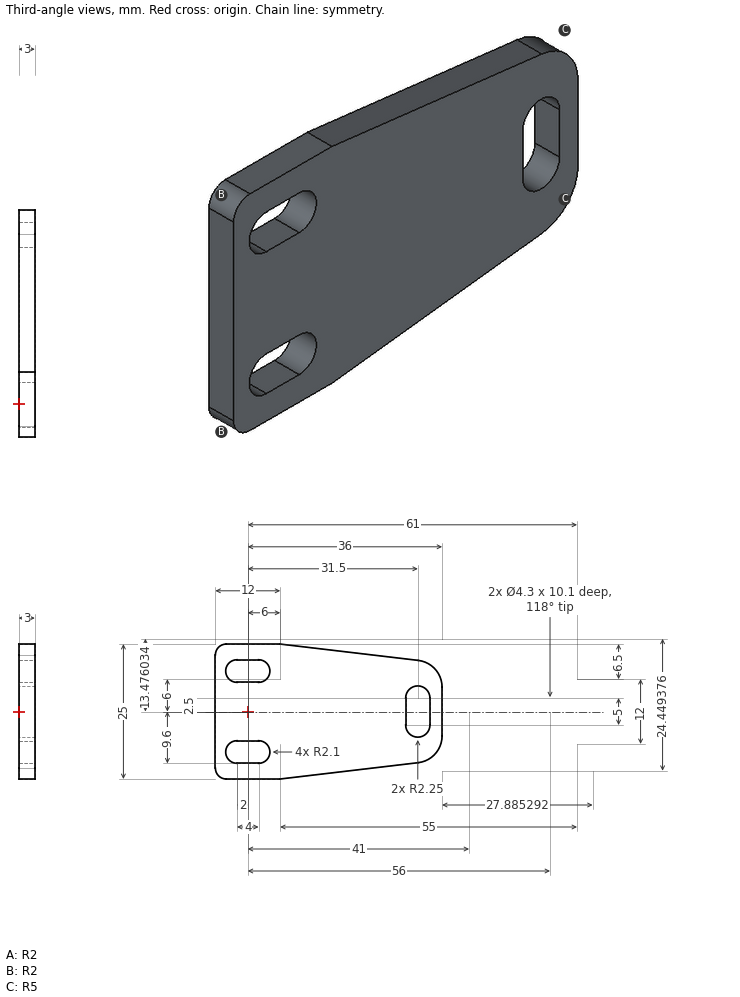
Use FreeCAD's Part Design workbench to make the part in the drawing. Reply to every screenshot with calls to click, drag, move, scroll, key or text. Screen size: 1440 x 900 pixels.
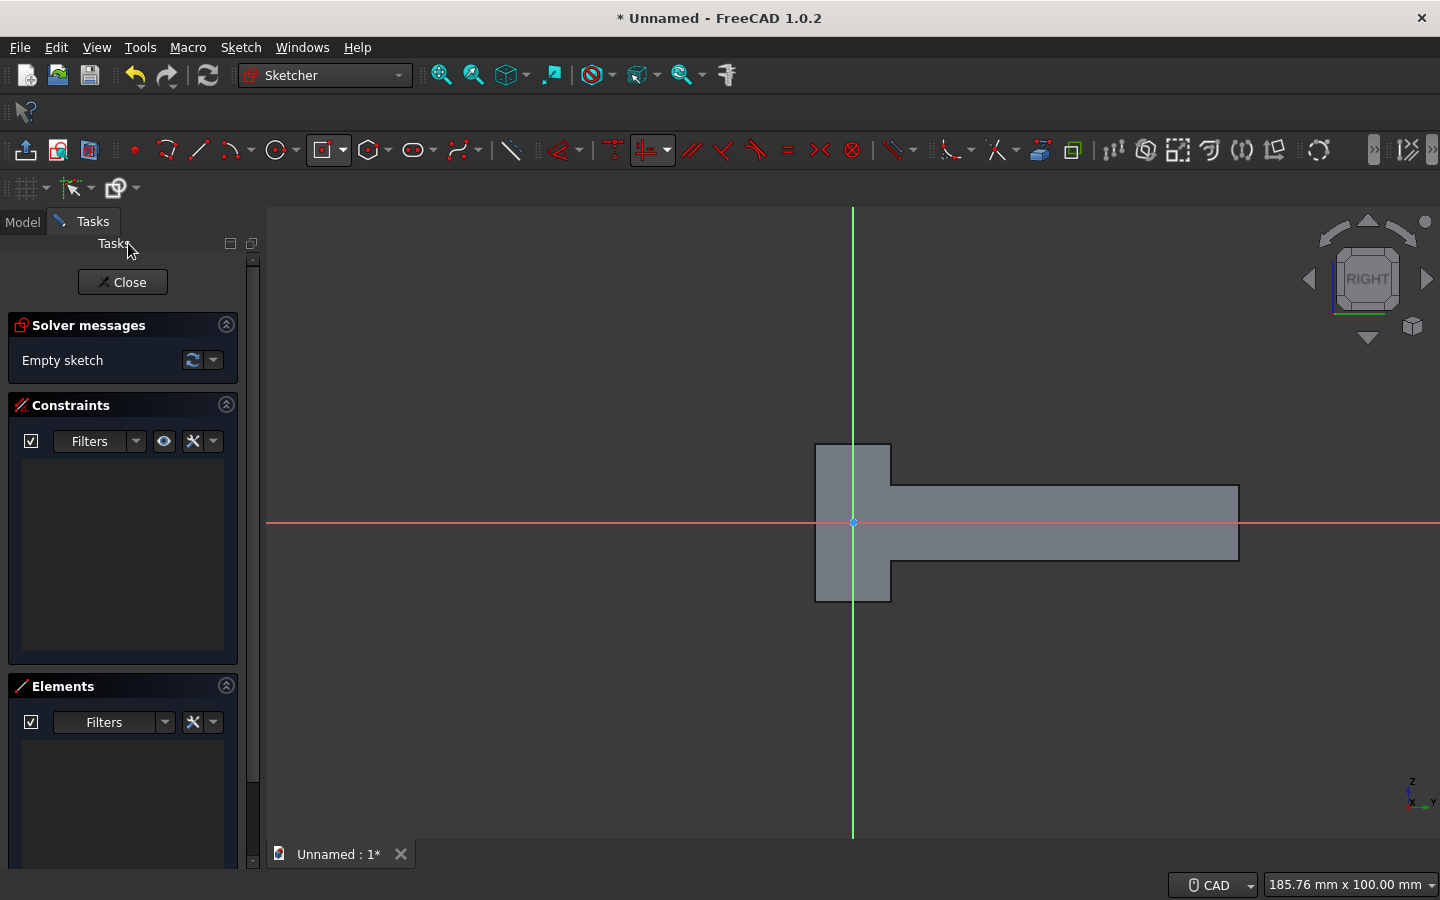
scroll(1275, 523, up, 3)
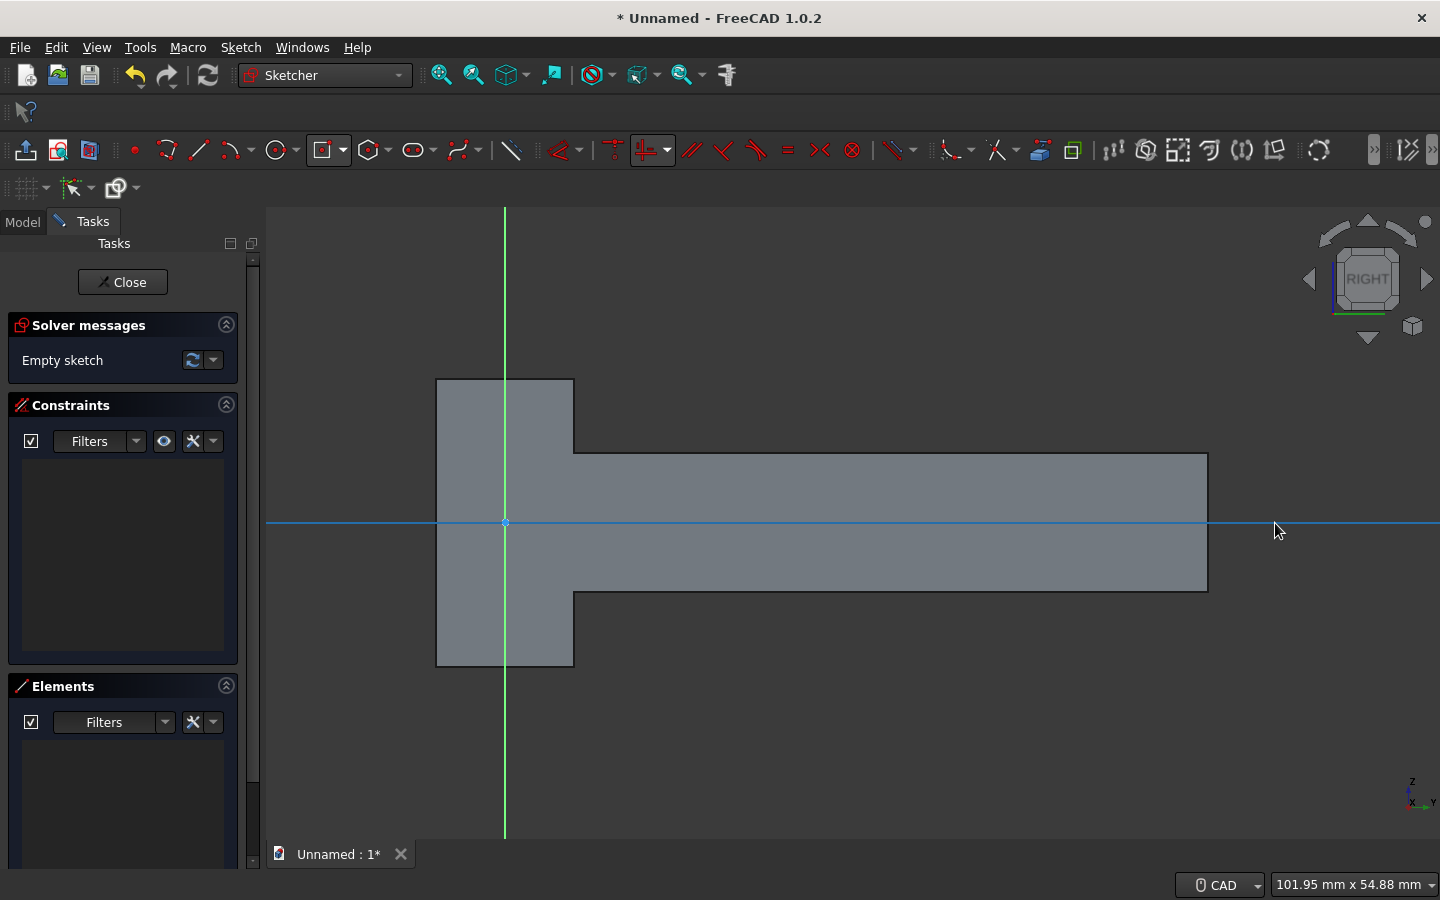
click(168, 150)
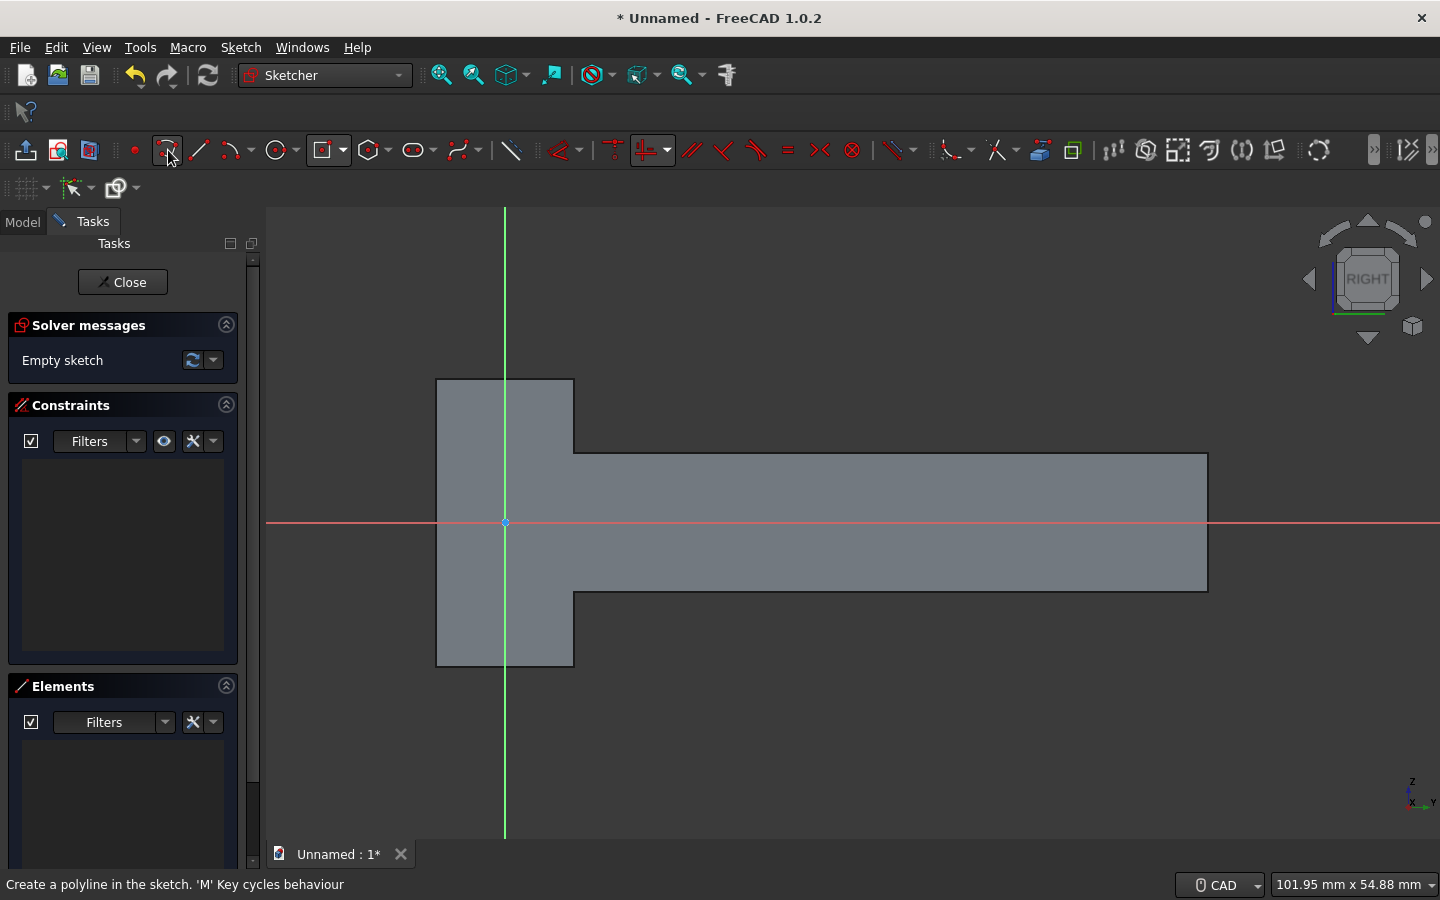
click(574, 667)
click(574, 379)
click(1208, 453)
click(1208, 592)
click(574, 668)
key(Escape)
key(Escape)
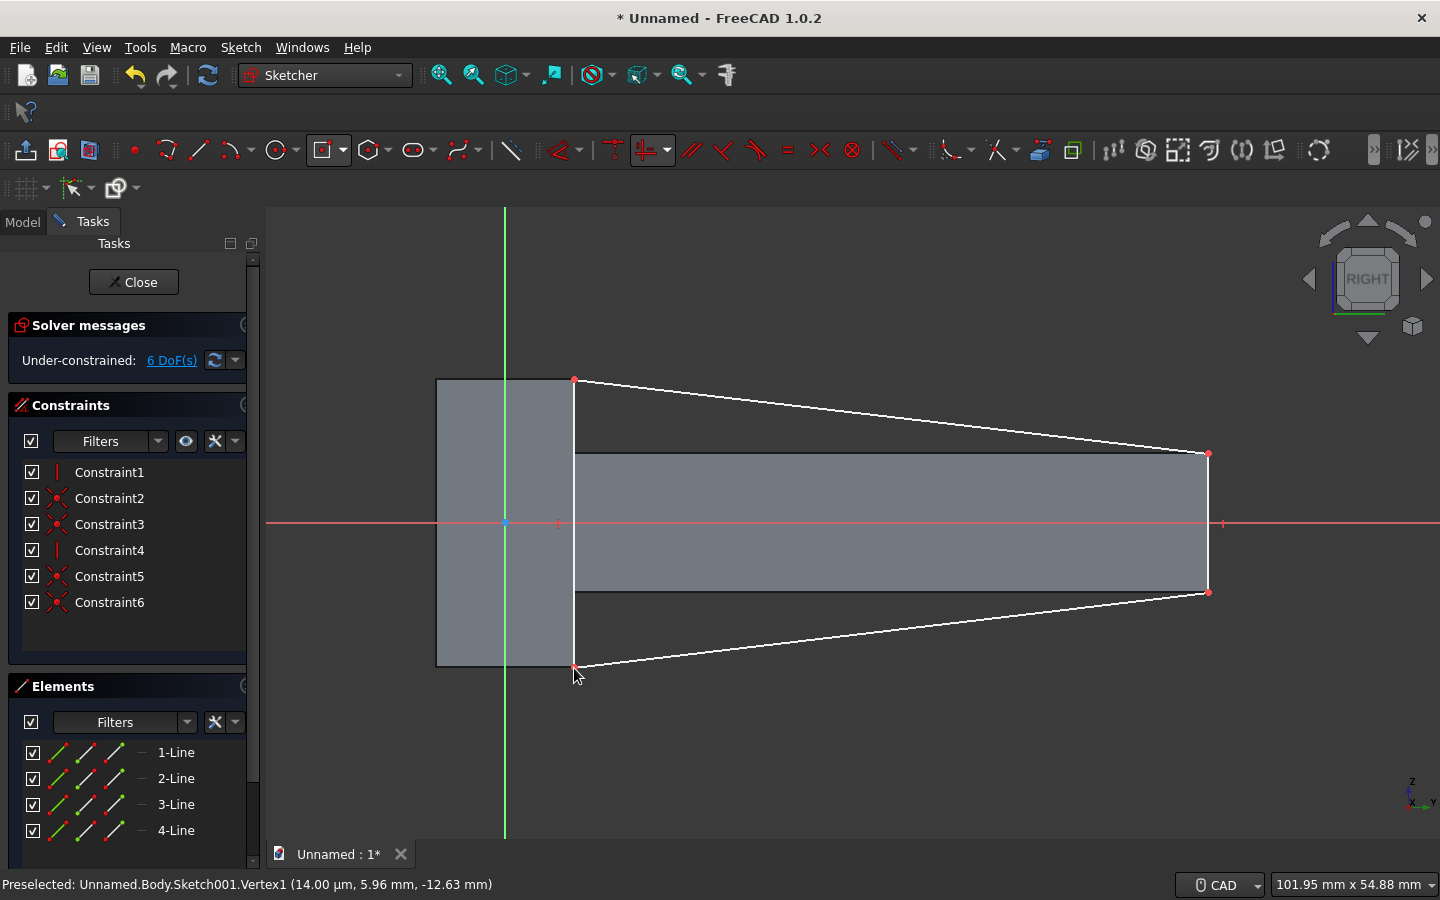
key(d)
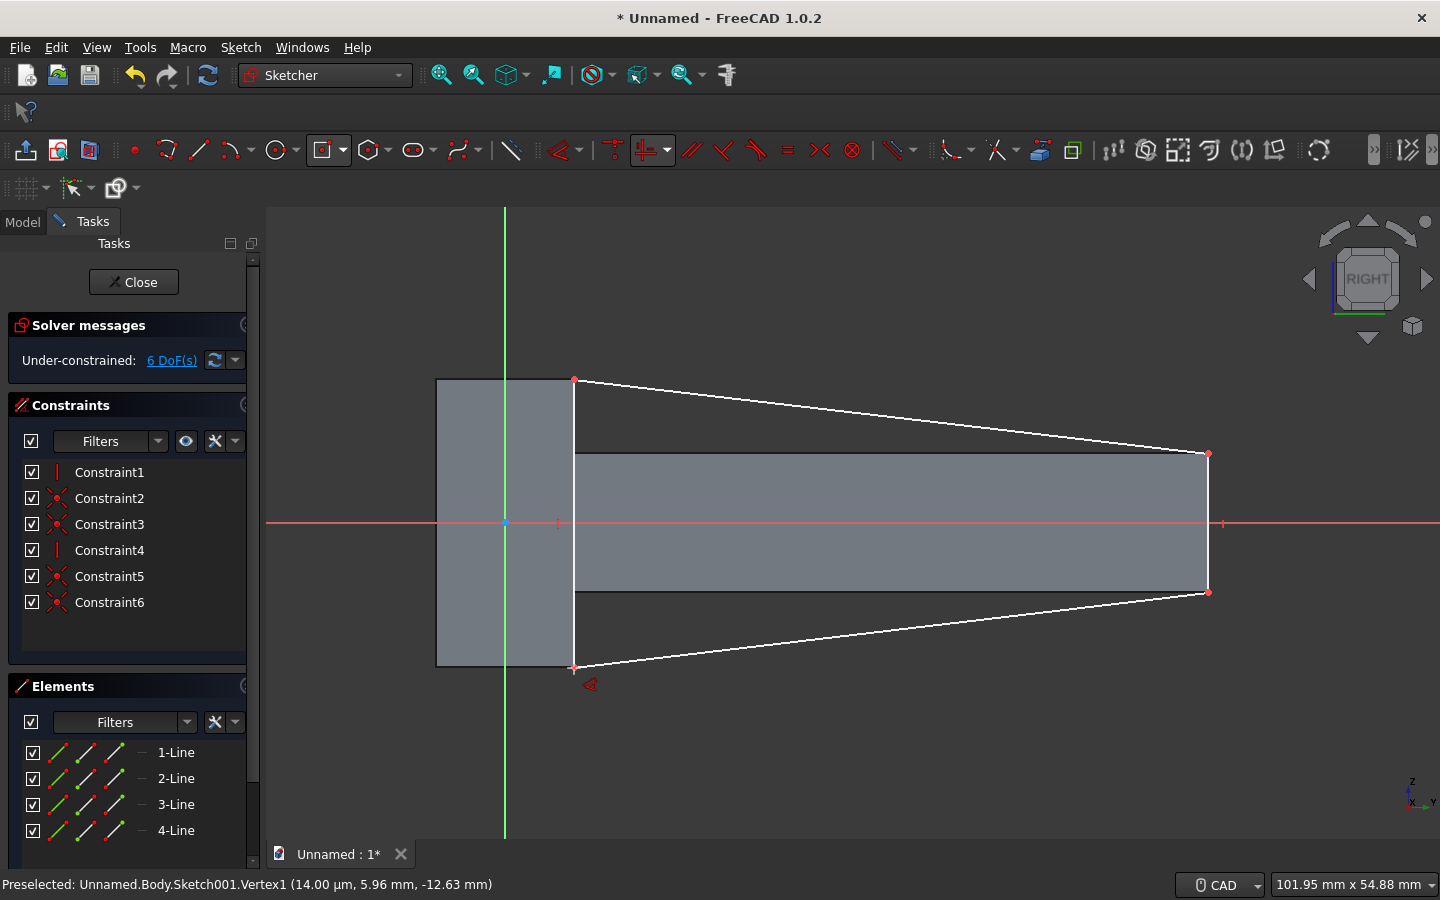
click(574, 582)
click(540, 458)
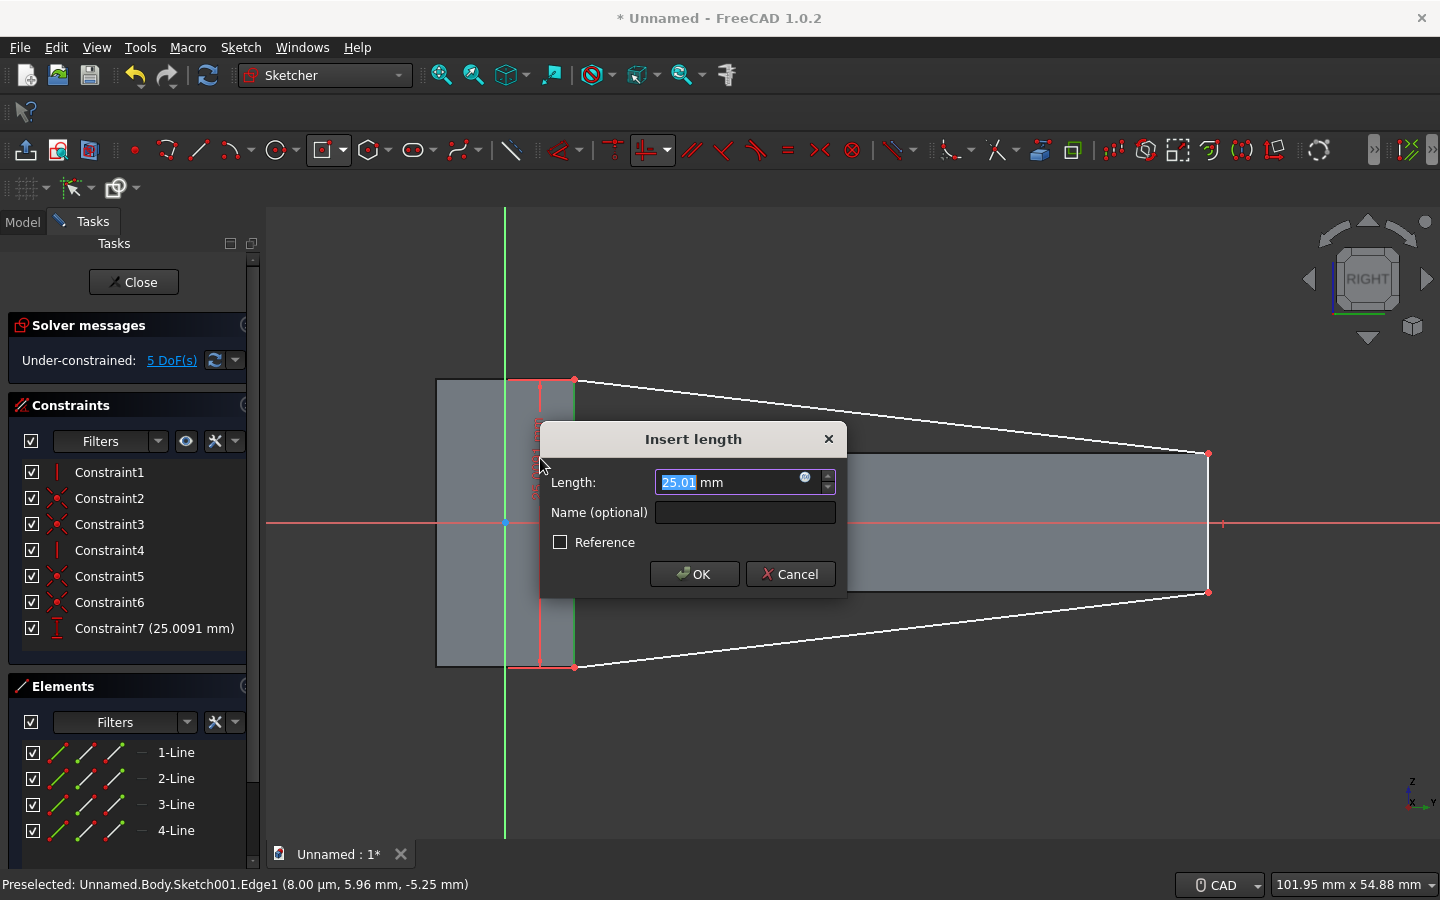
text(25)
key(Return)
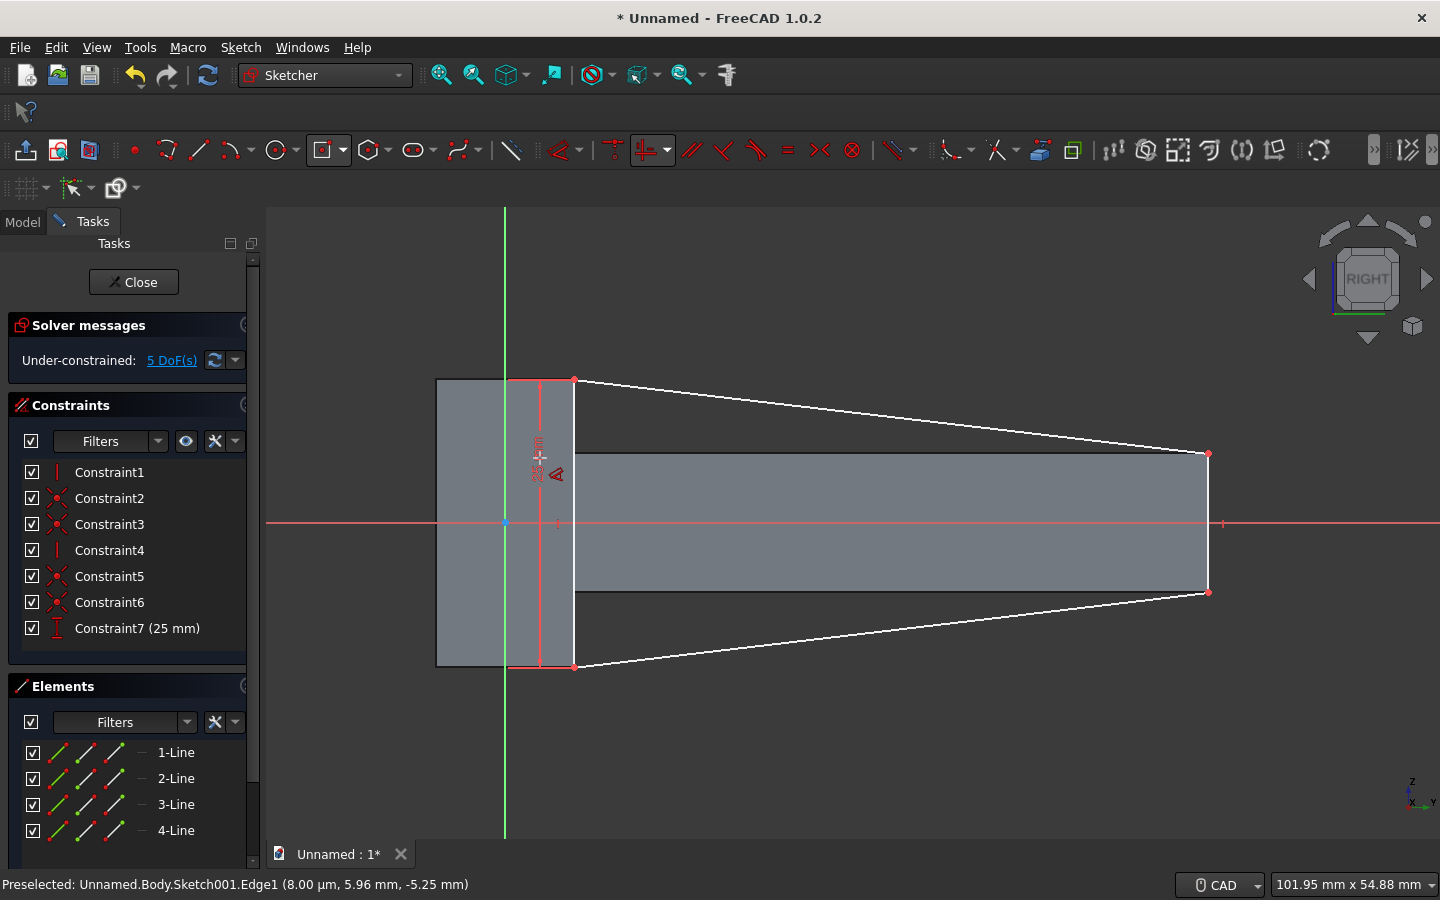
click(1208, 496)
click(1242, 492)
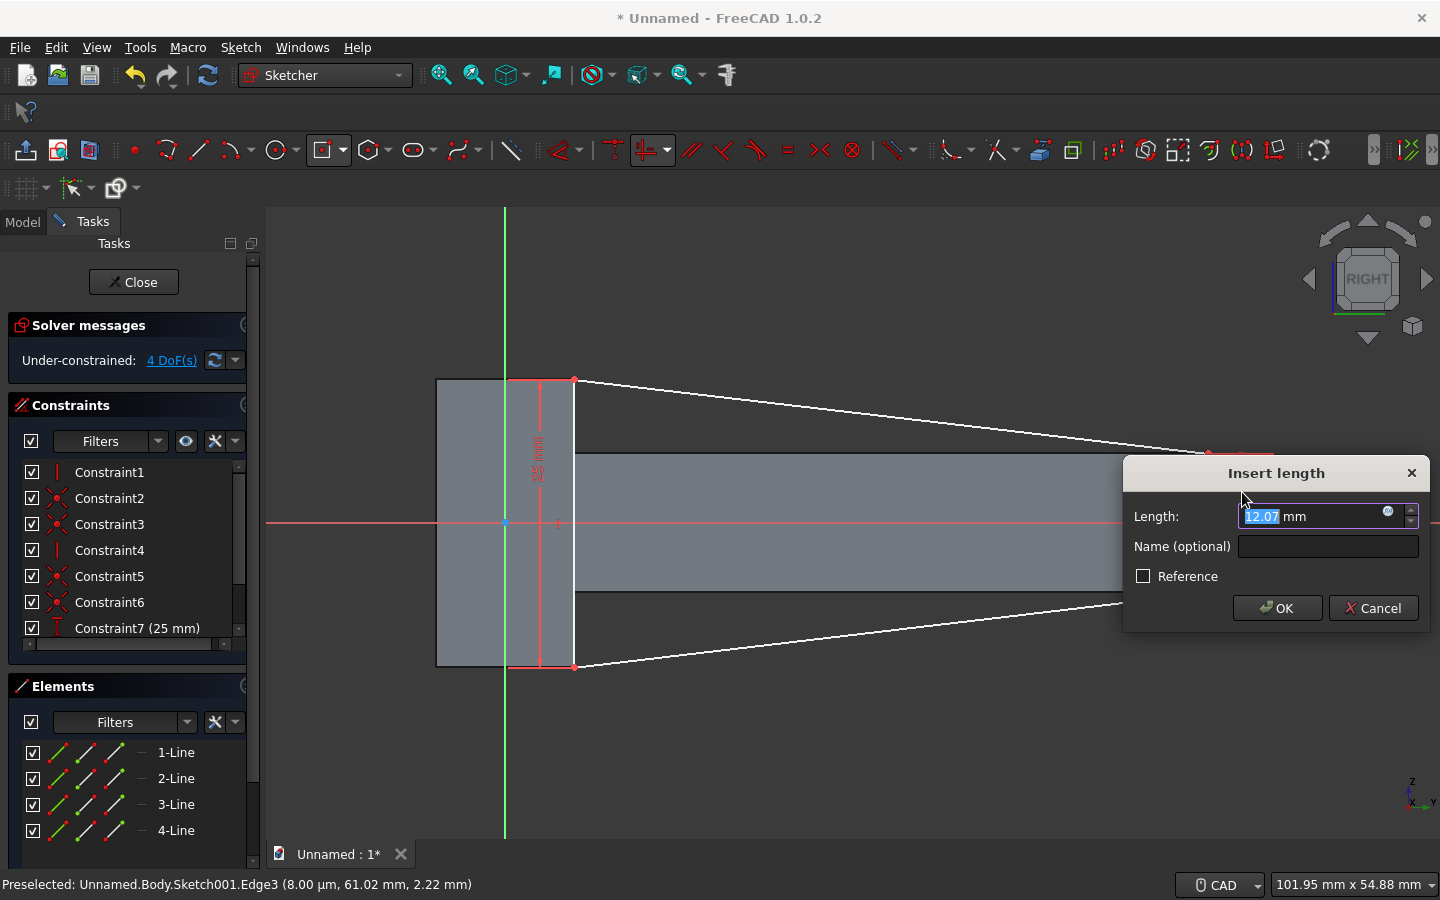
text(12)
key(Return)